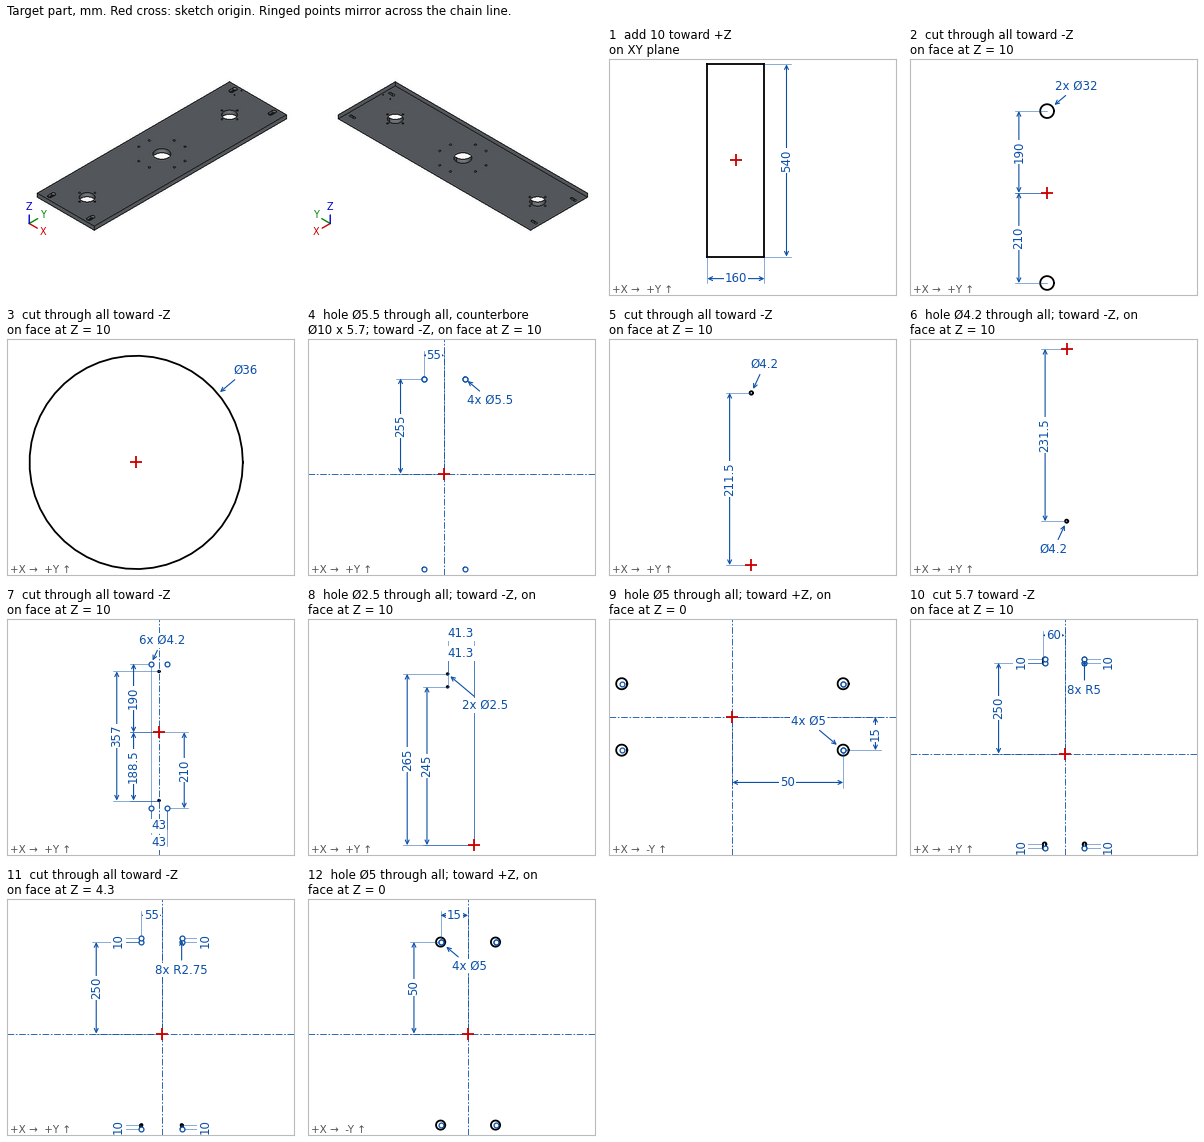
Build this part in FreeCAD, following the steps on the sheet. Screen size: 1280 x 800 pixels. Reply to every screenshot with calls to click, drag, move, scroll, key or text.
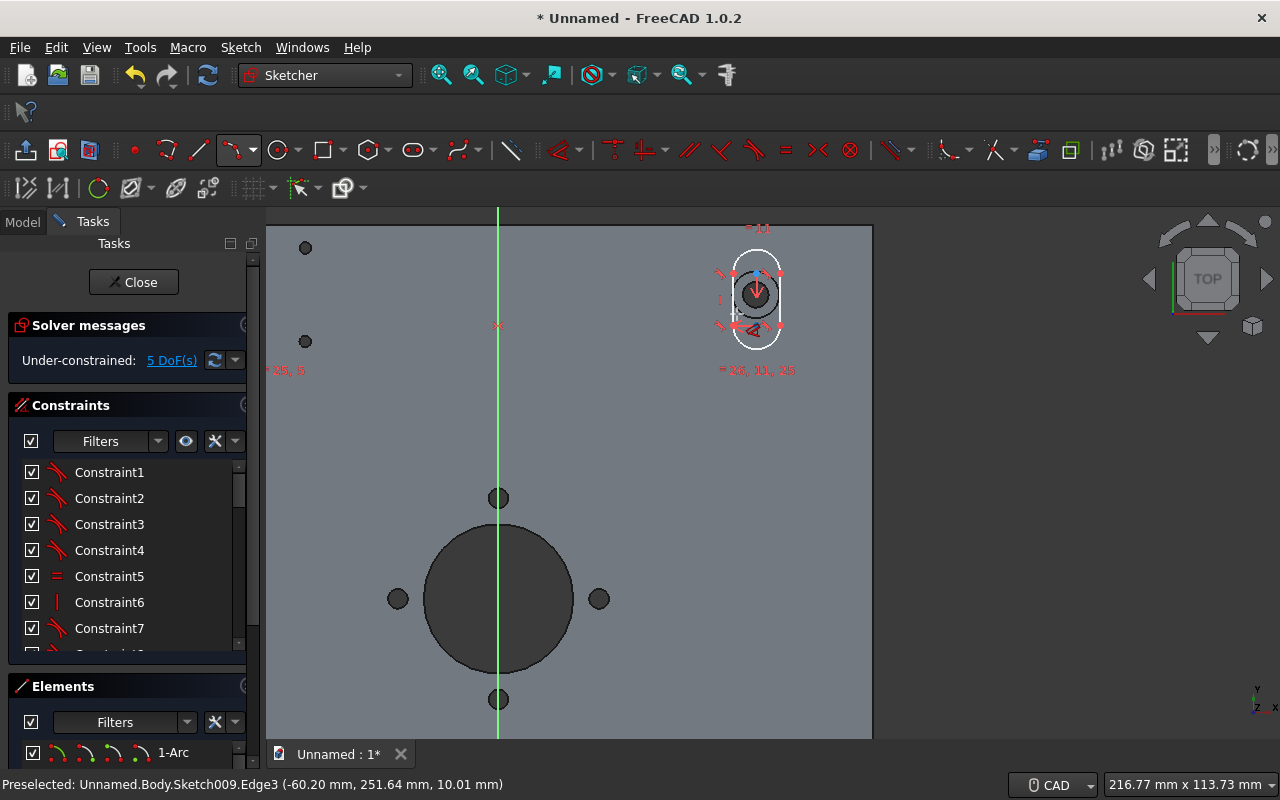
click(733, 310)
click(699, 299)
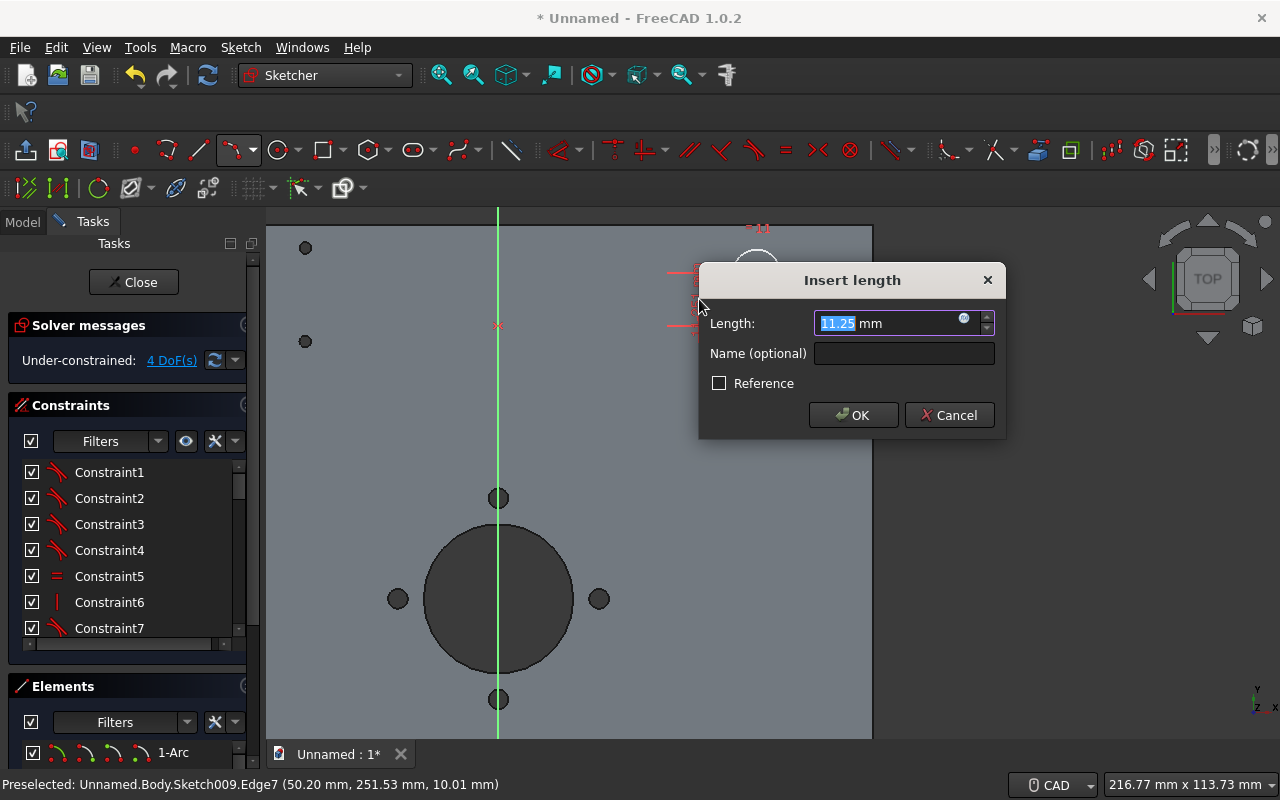
text(10)
key(Return)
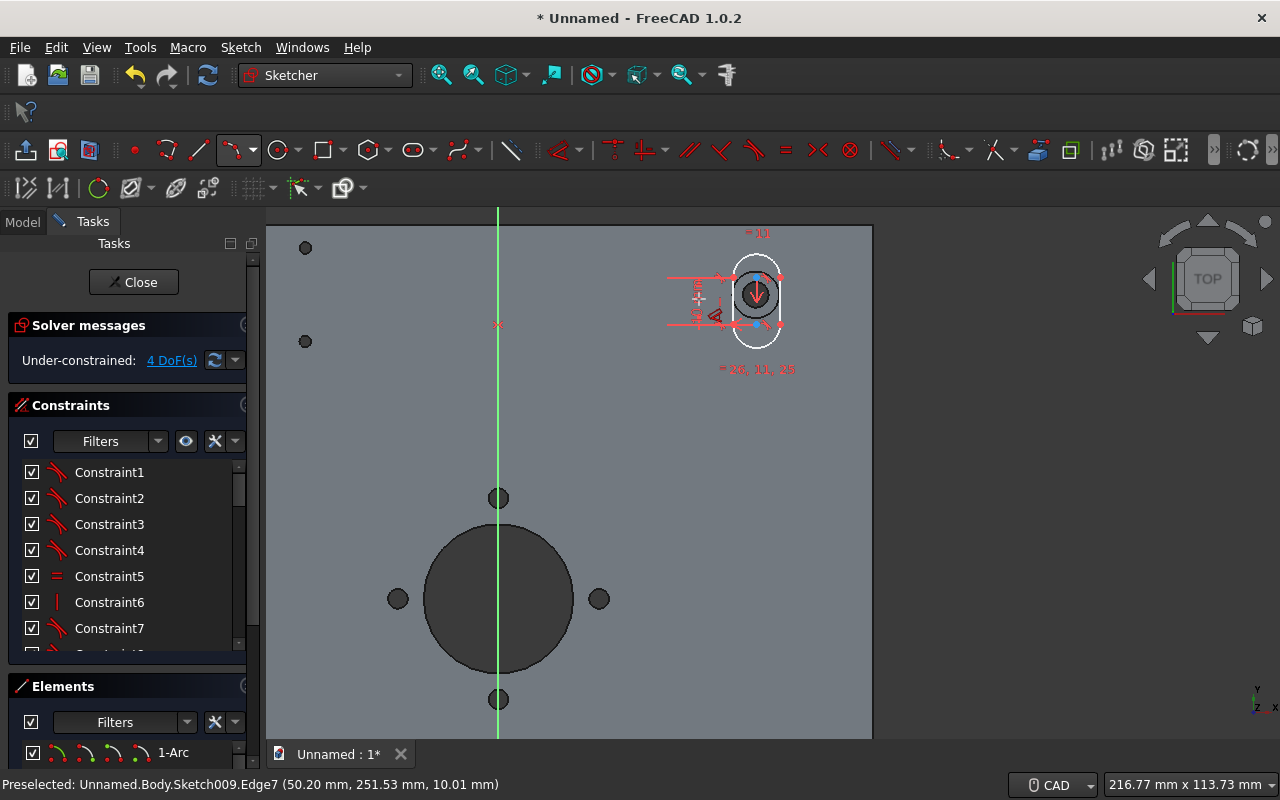
scroll(737, 314, down, 10)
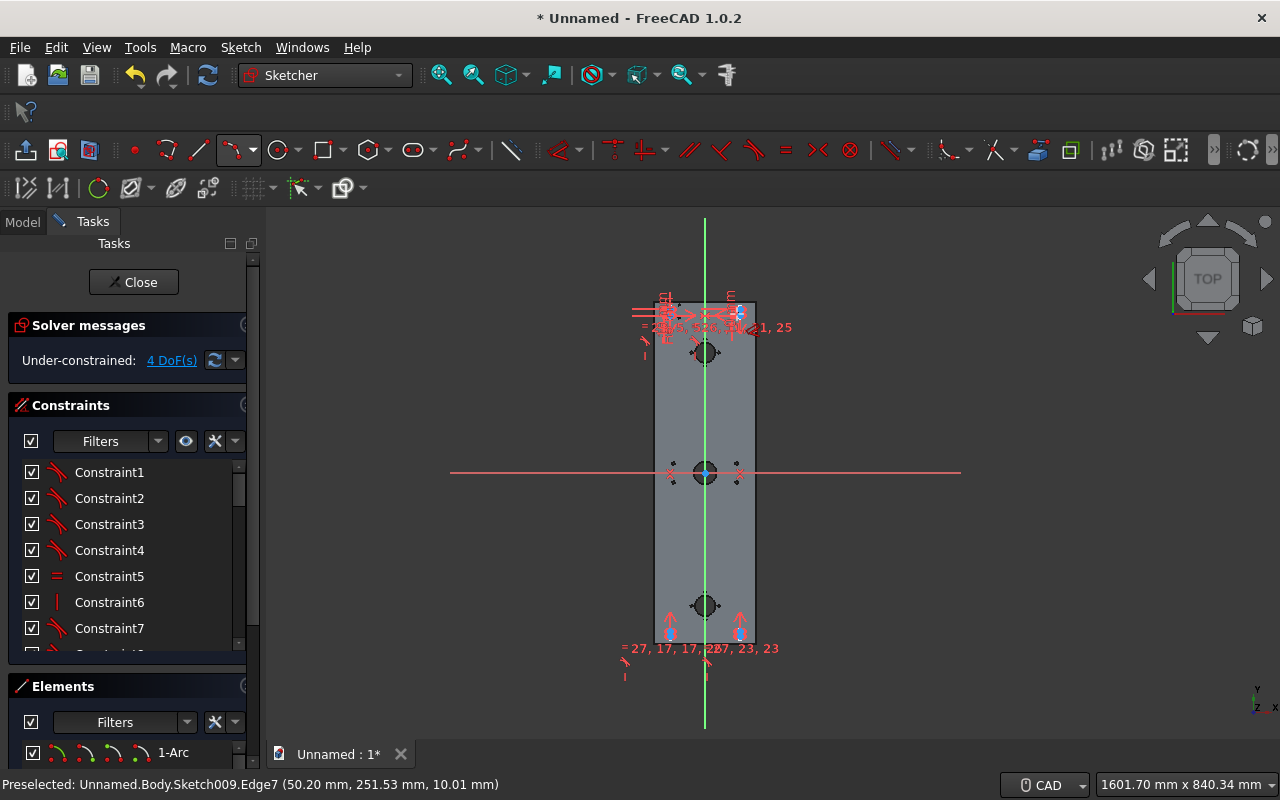
scroll(667, 635, up, 12)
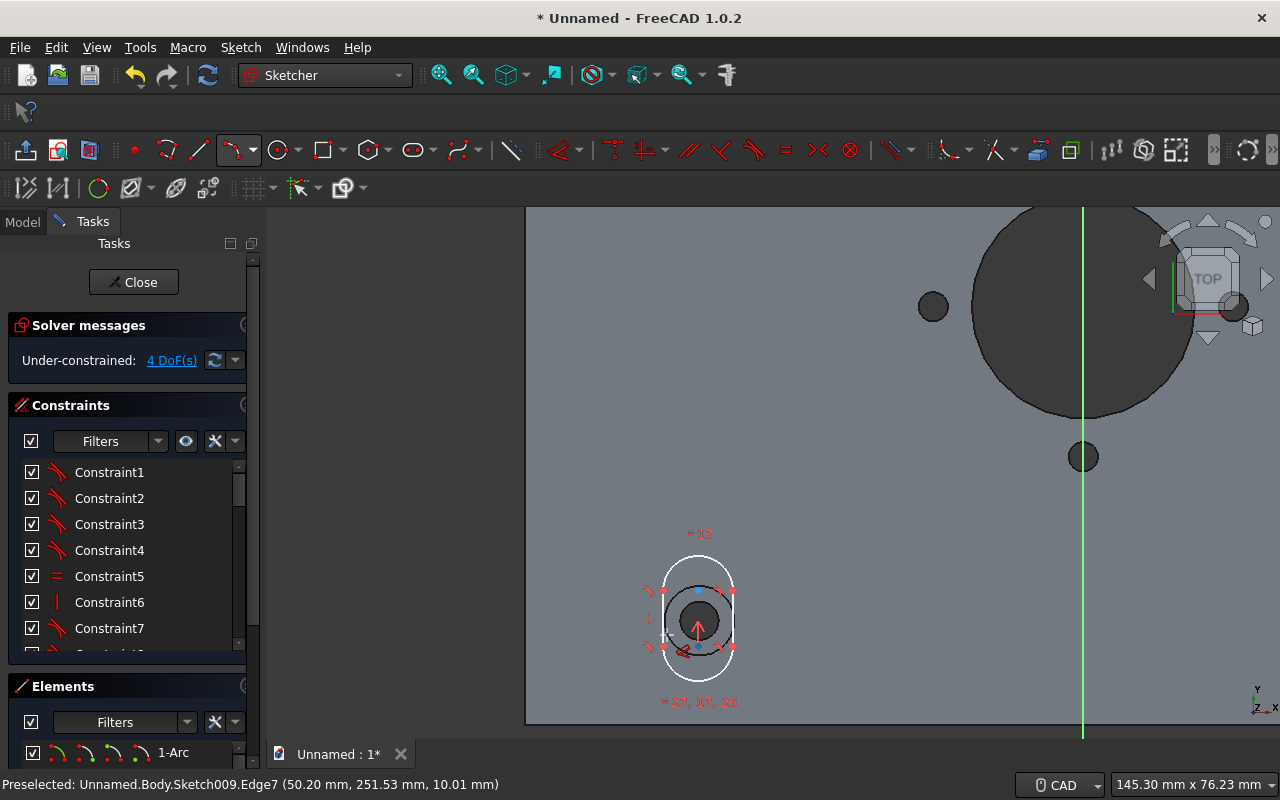
click(663, 630)
click(629, 619)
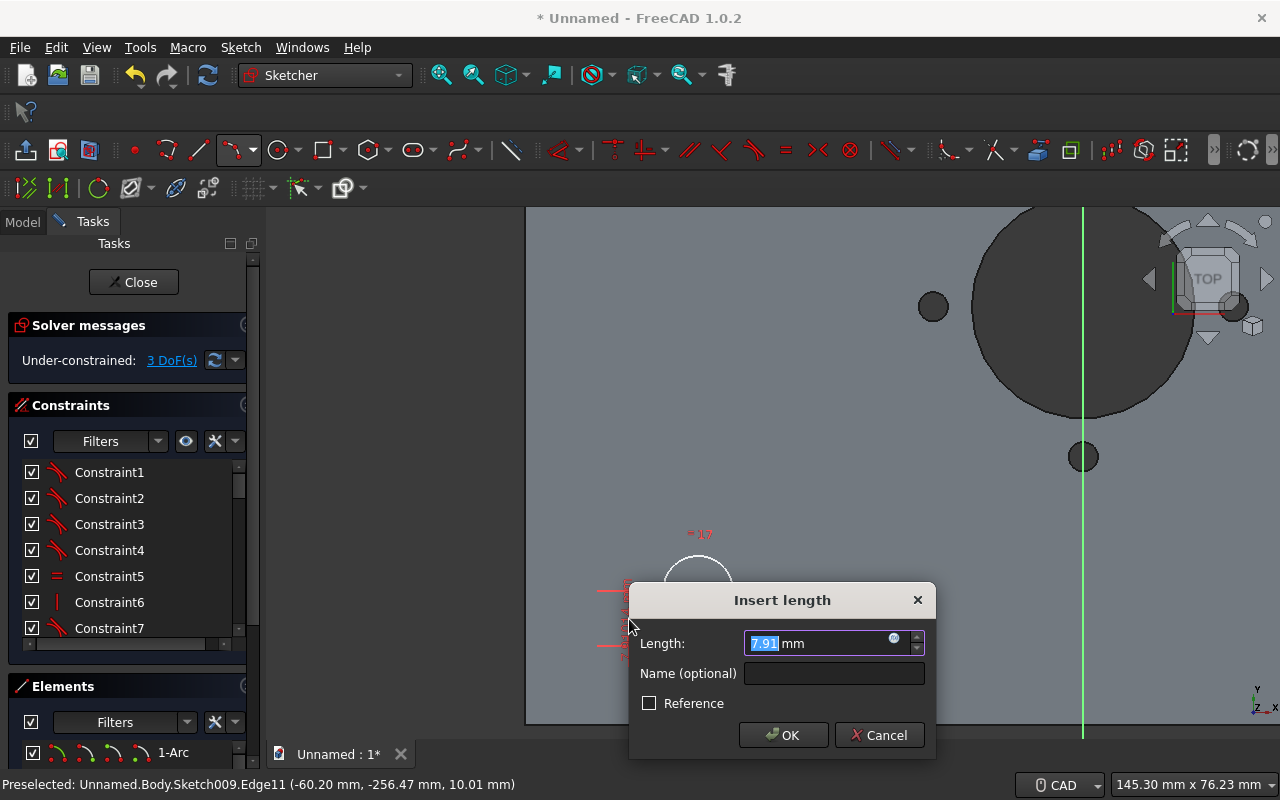
text(10)
key(Return)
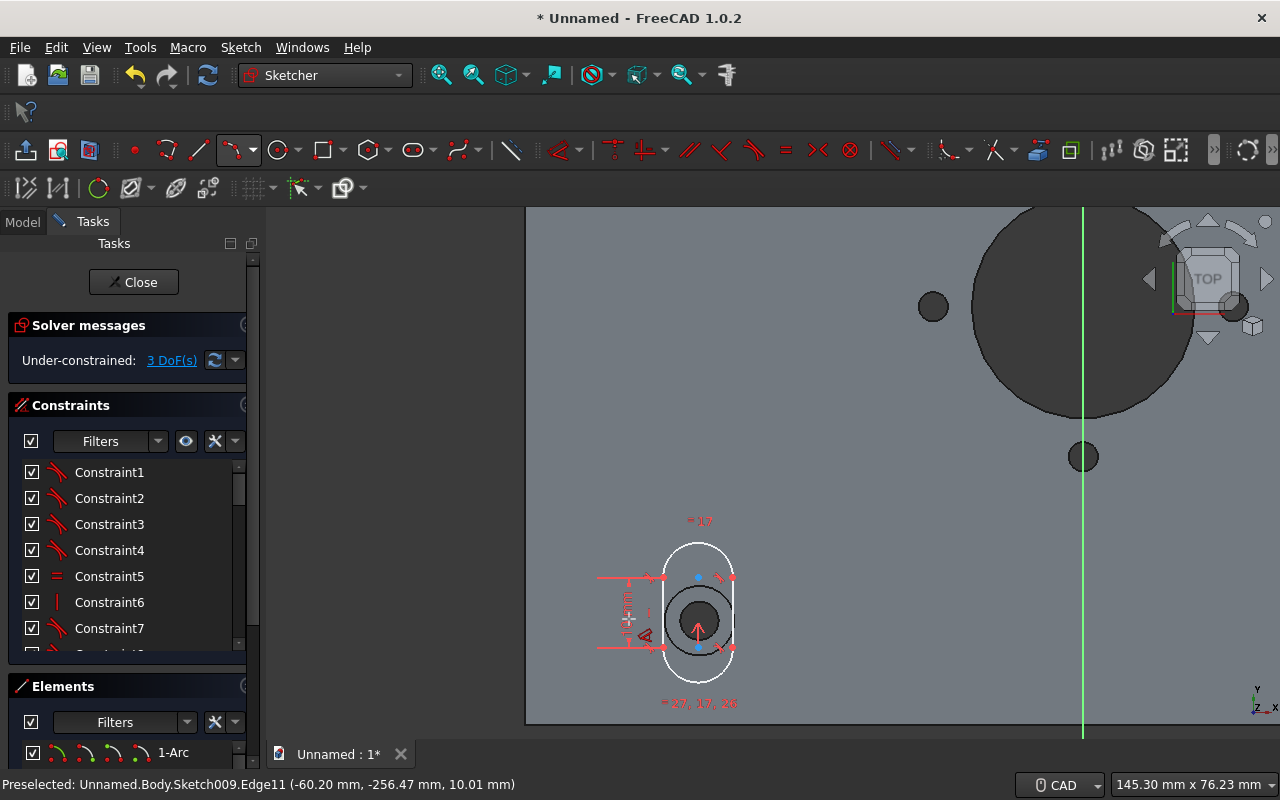
scroll(667, 636, down, 12)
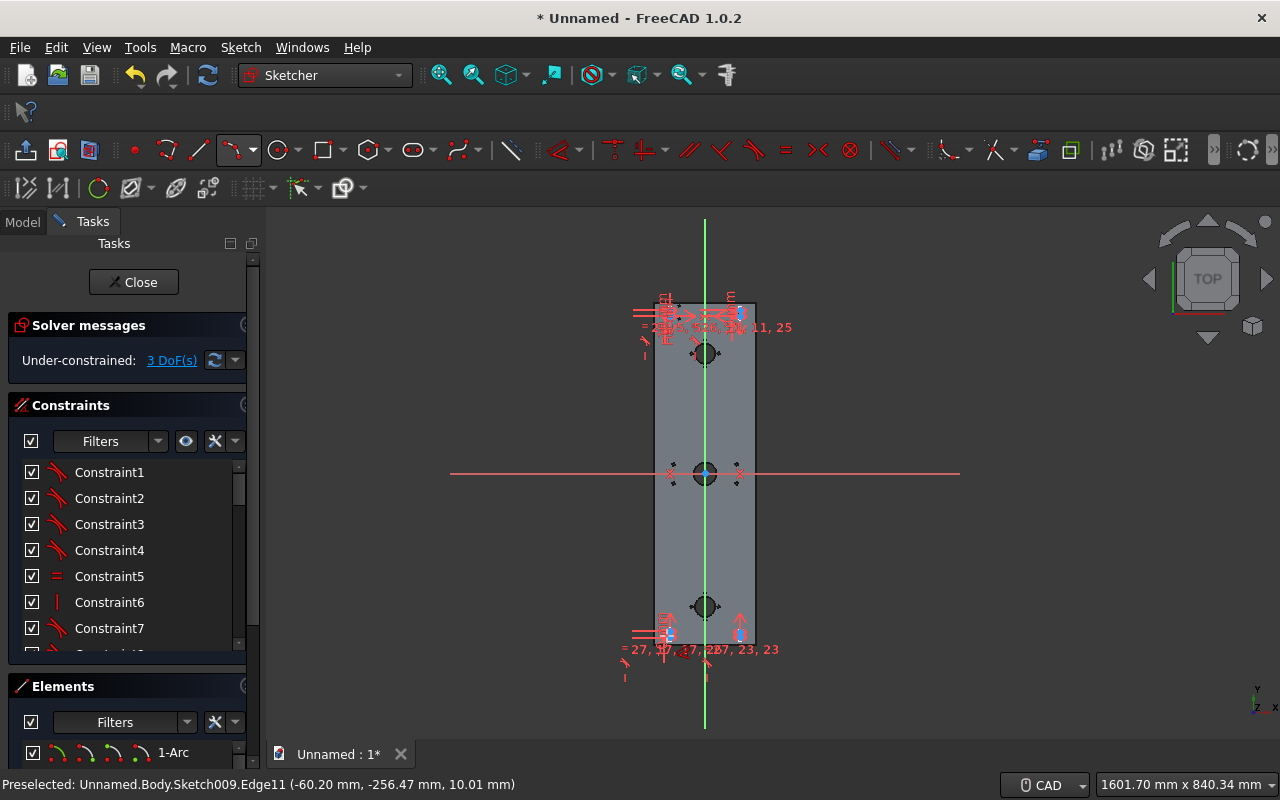
scroll(737, 636, up, 12)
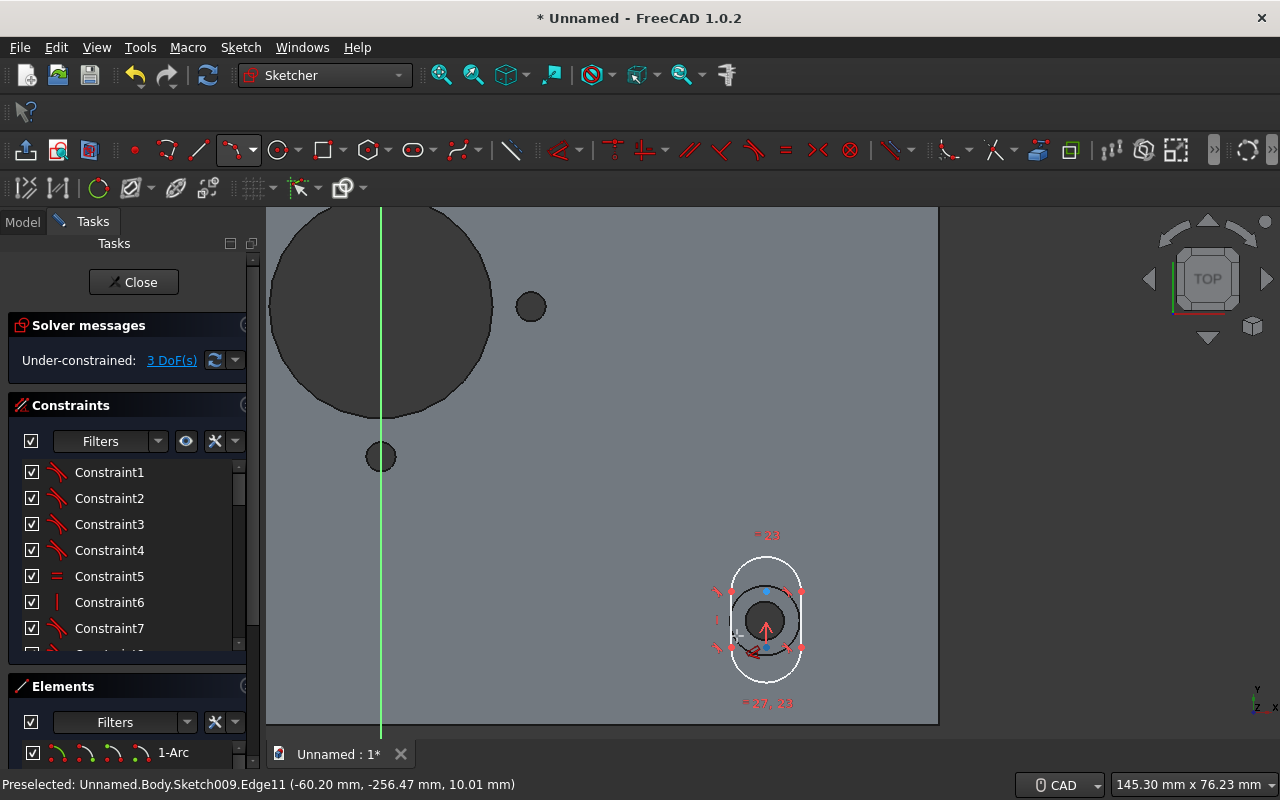
click(731, 631)
click(765, 620)